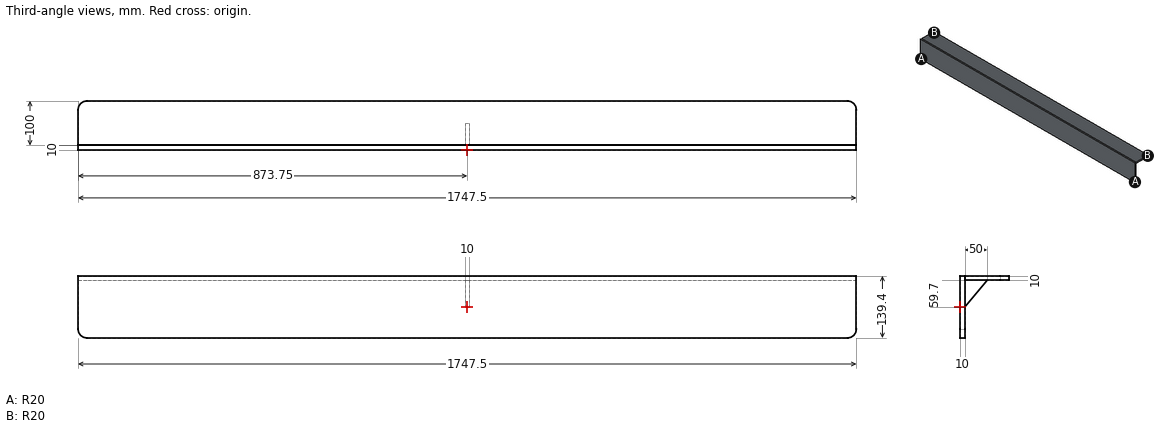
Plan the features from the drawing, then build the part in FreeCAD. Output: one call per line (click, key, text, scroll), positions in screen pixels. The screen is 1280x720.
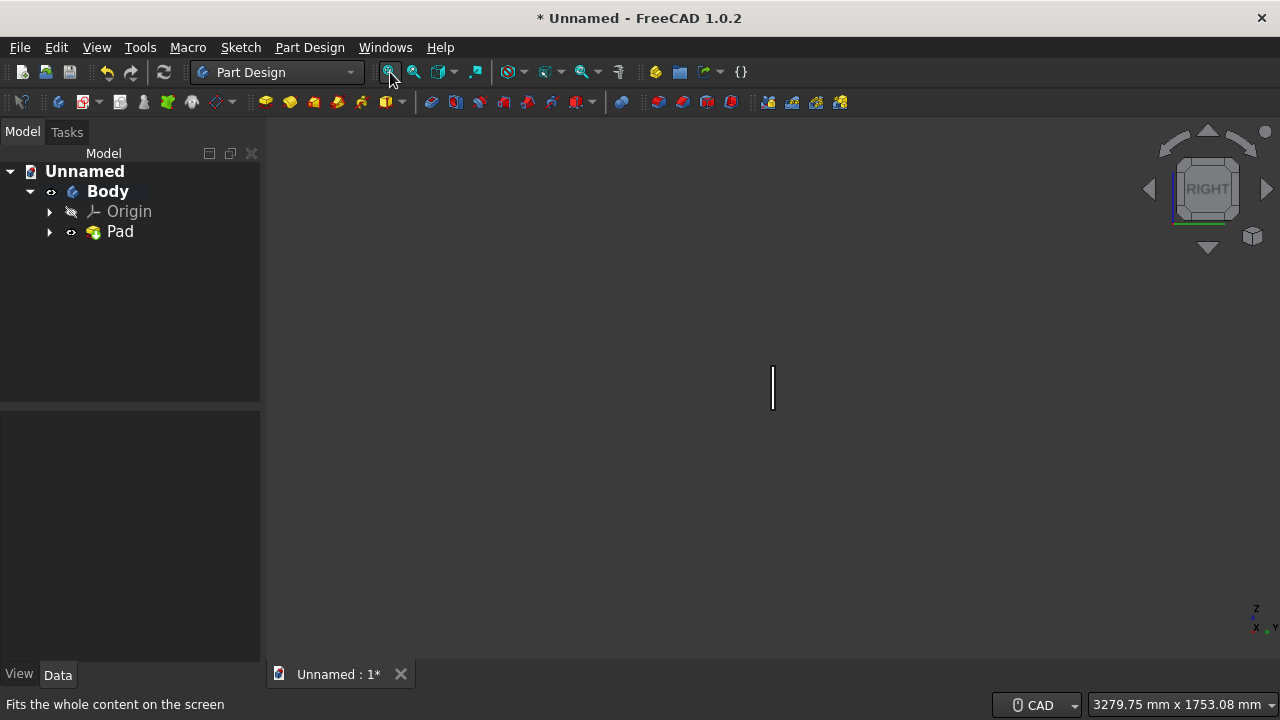
scroll(773, 409, up, 13)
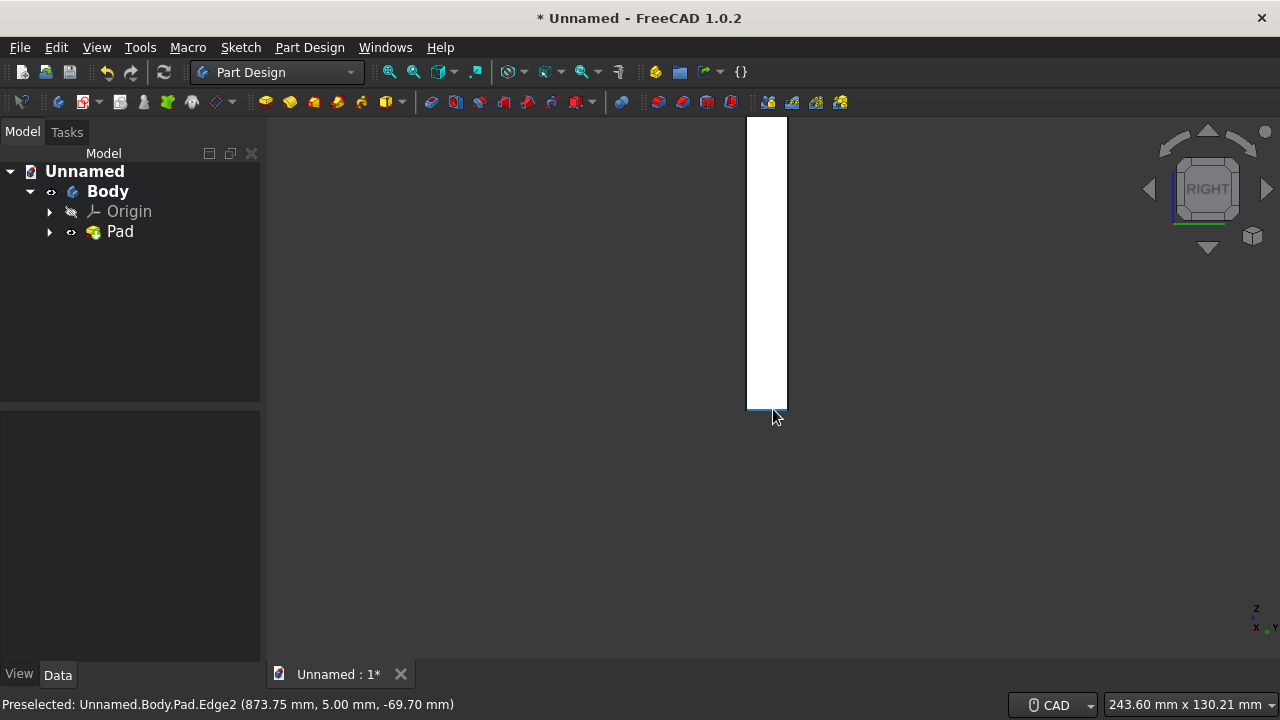
click(767, 409)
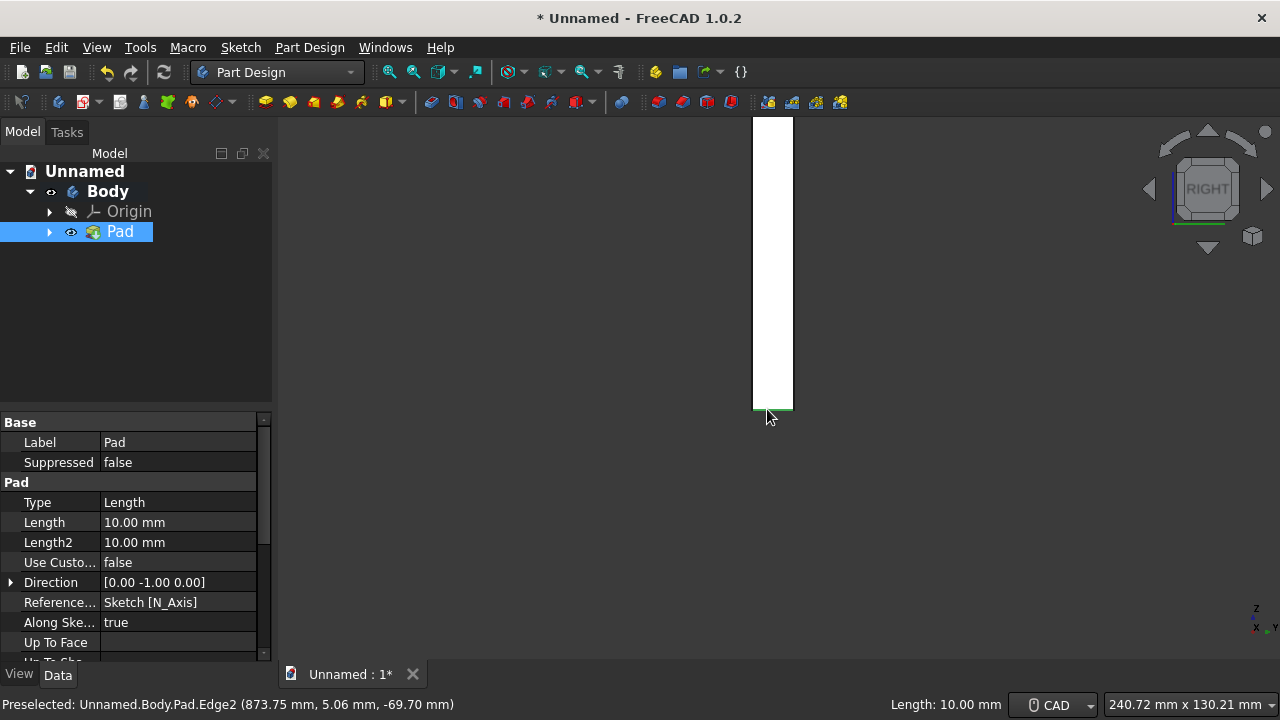
click(390, 72)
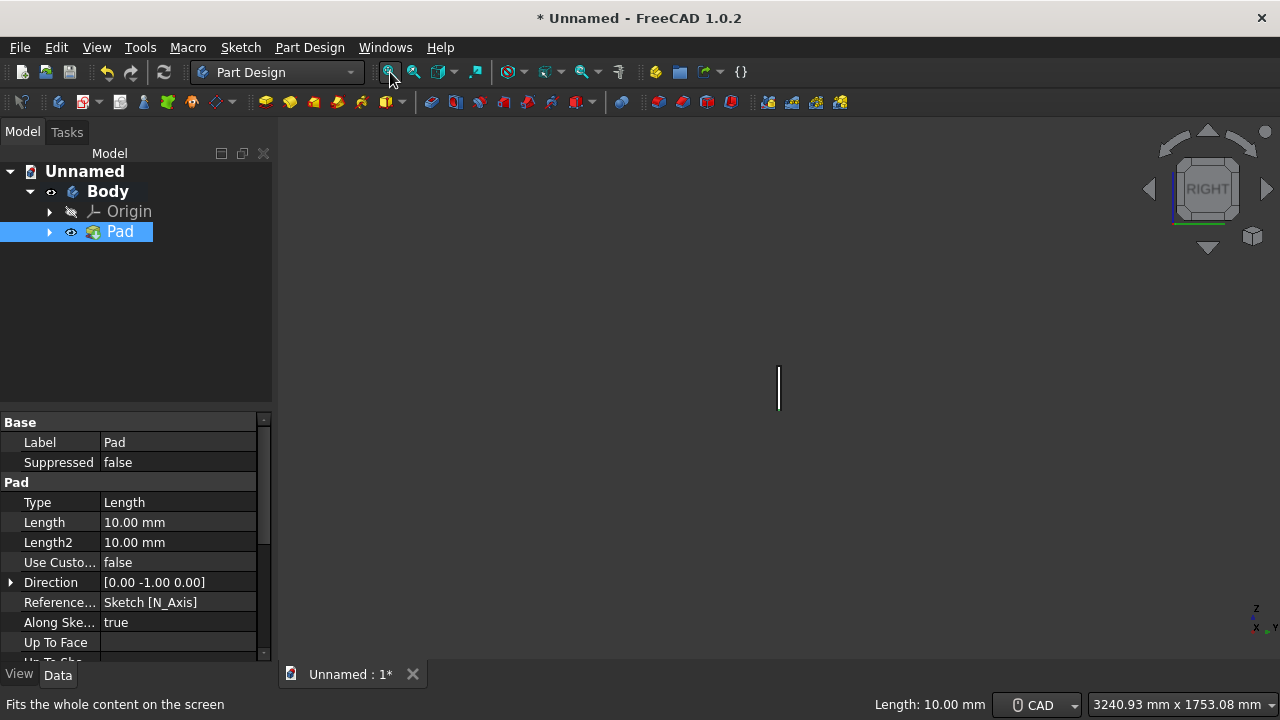
key(5)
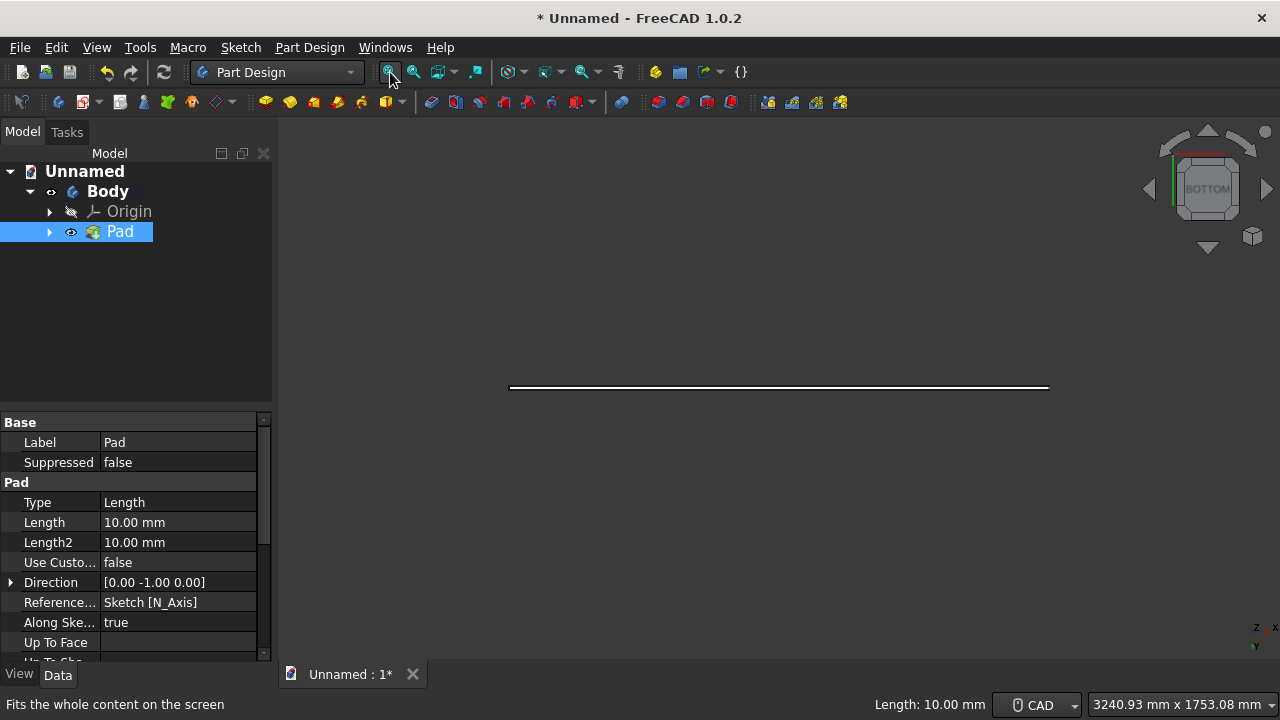
scroll(509, 387, up, 13)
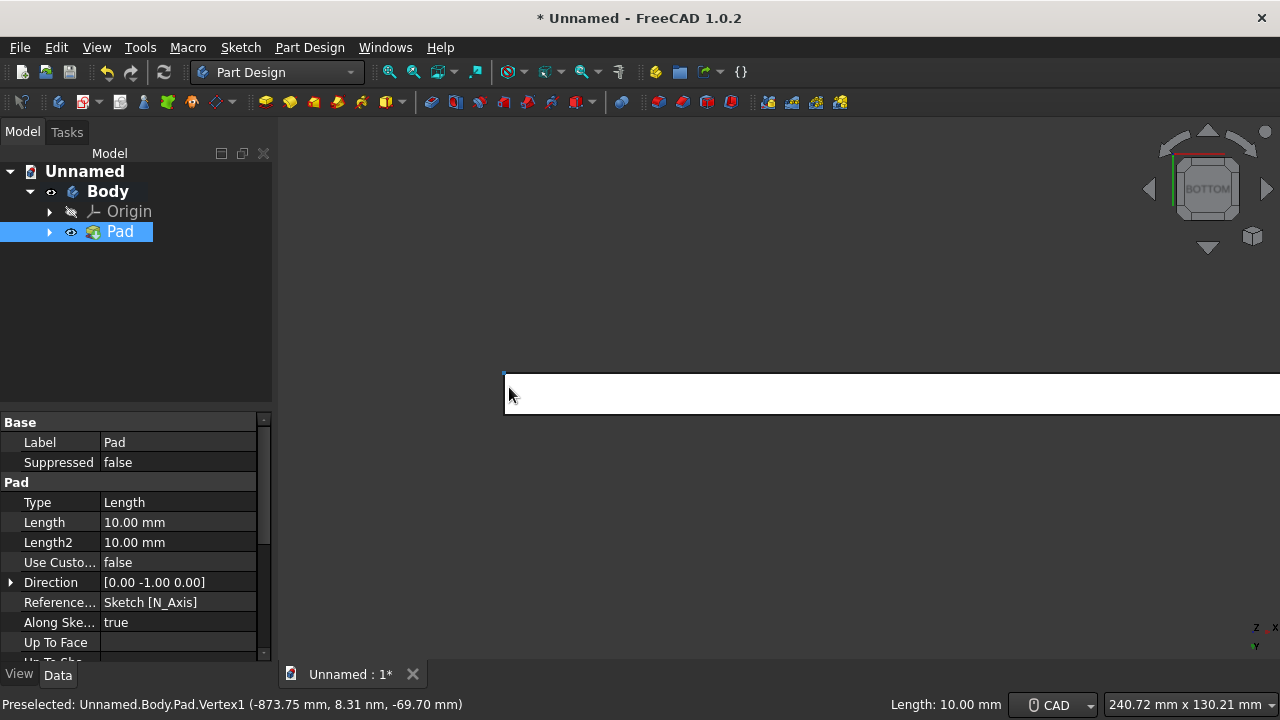
click(504, 393, ctrl)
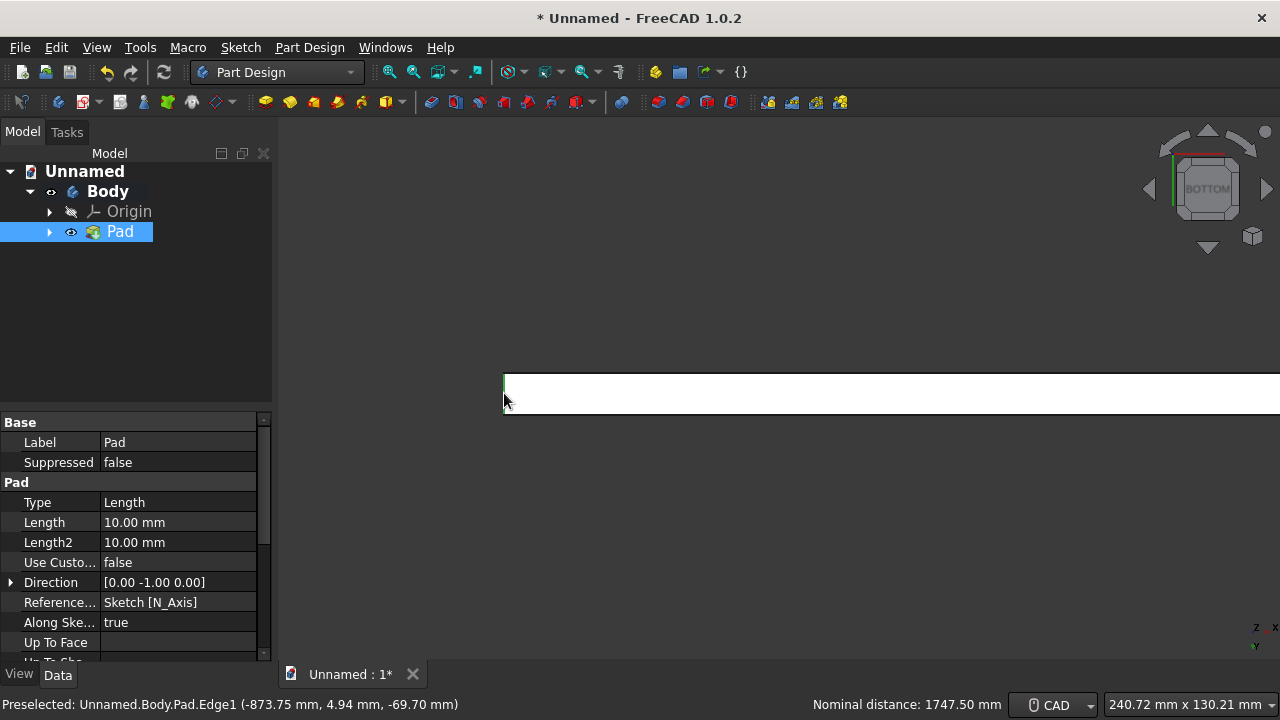
click(660, 102)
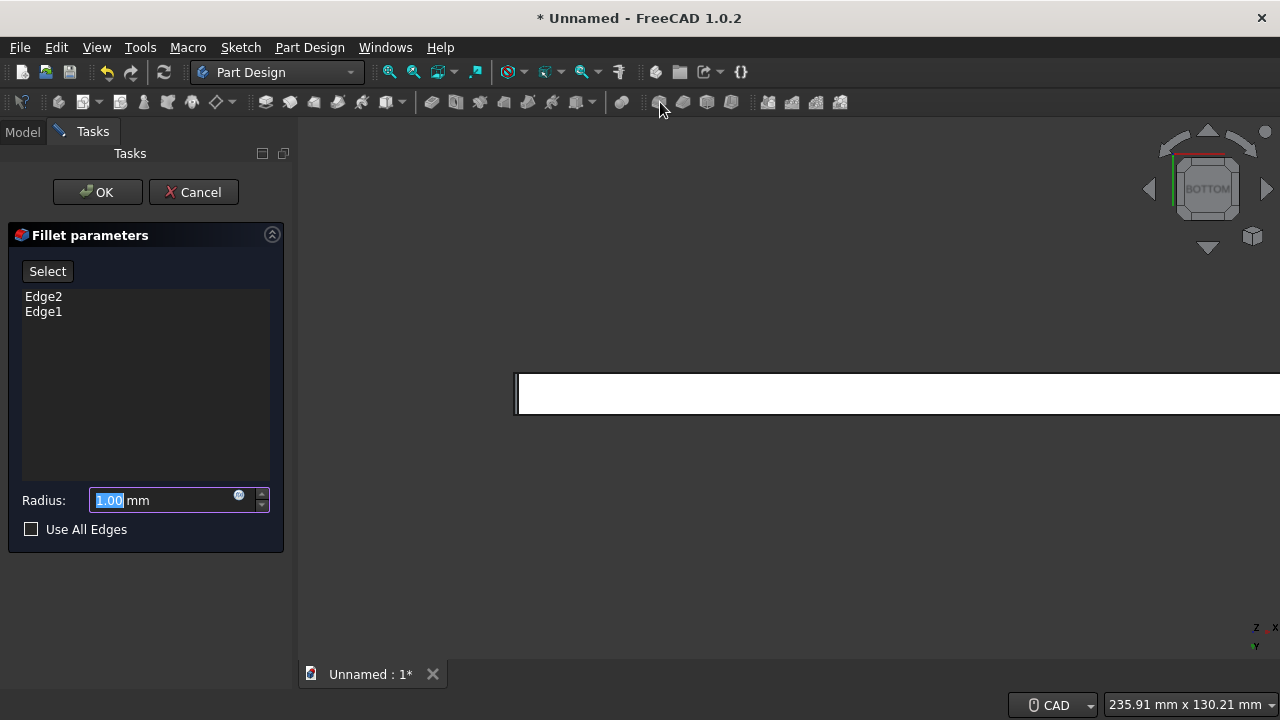
text(20)
key(Tab)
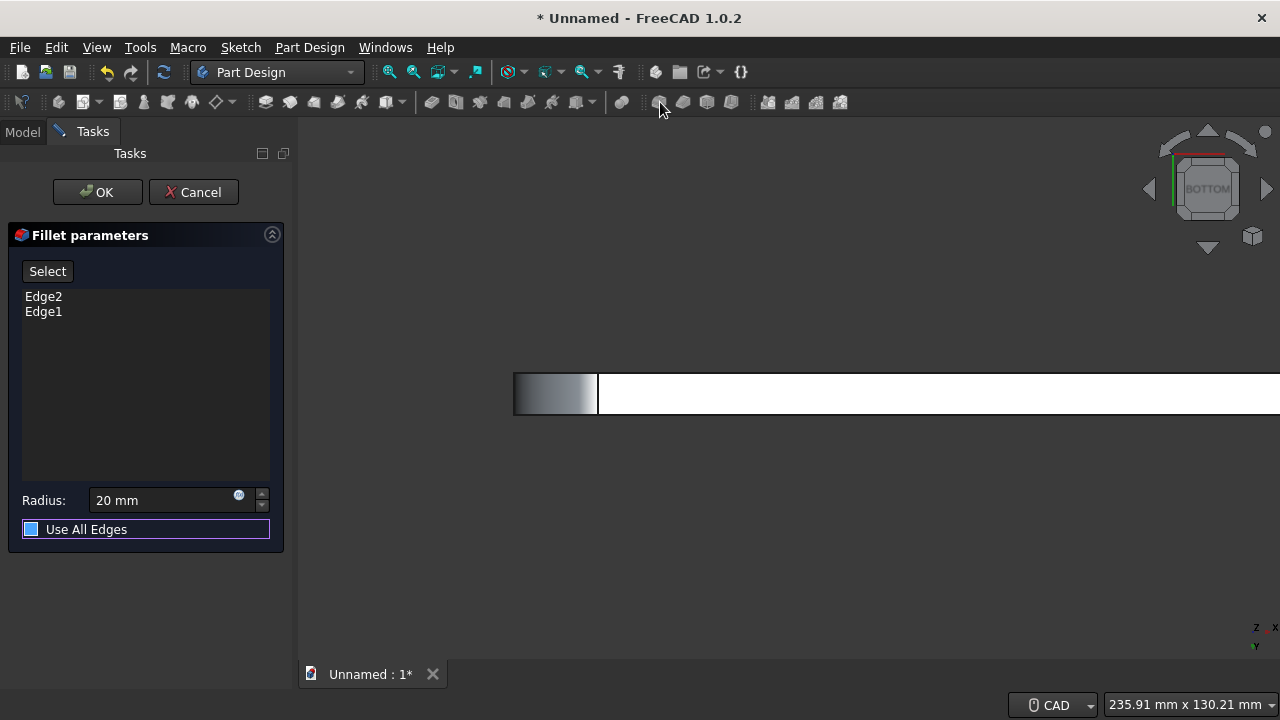
click(98, 192)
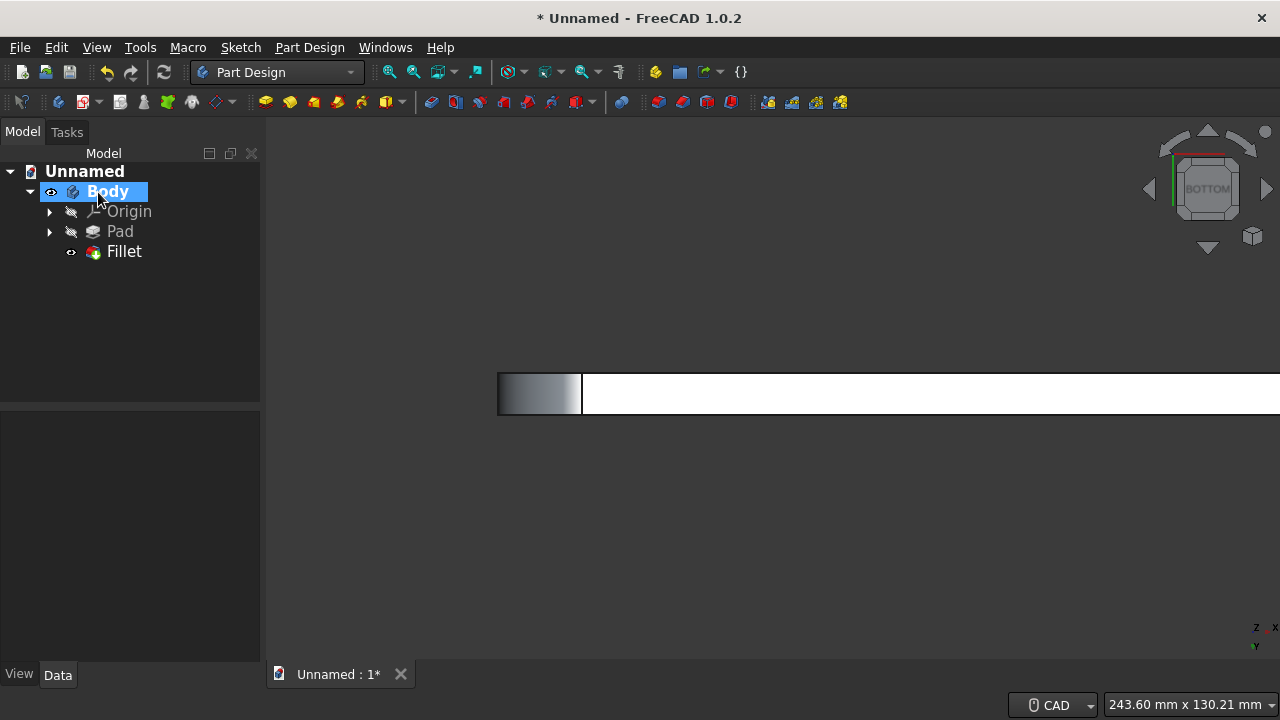
click(390, 72)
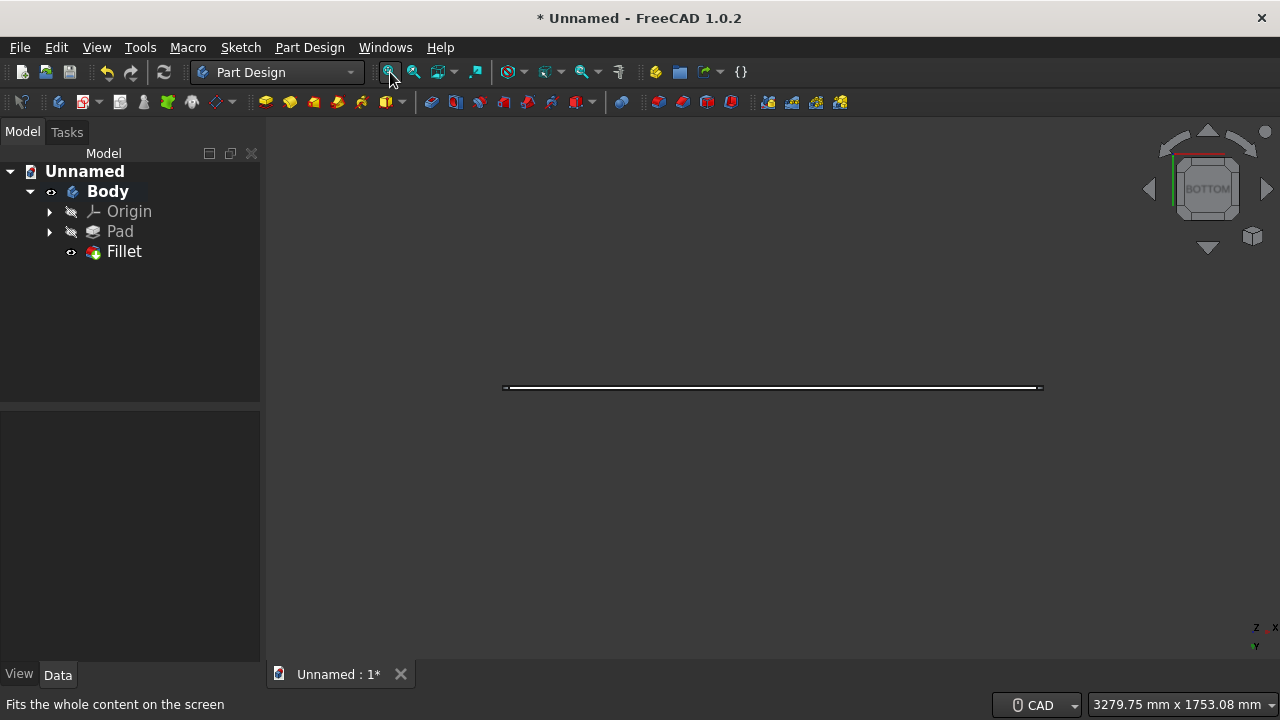
click(60, 102)